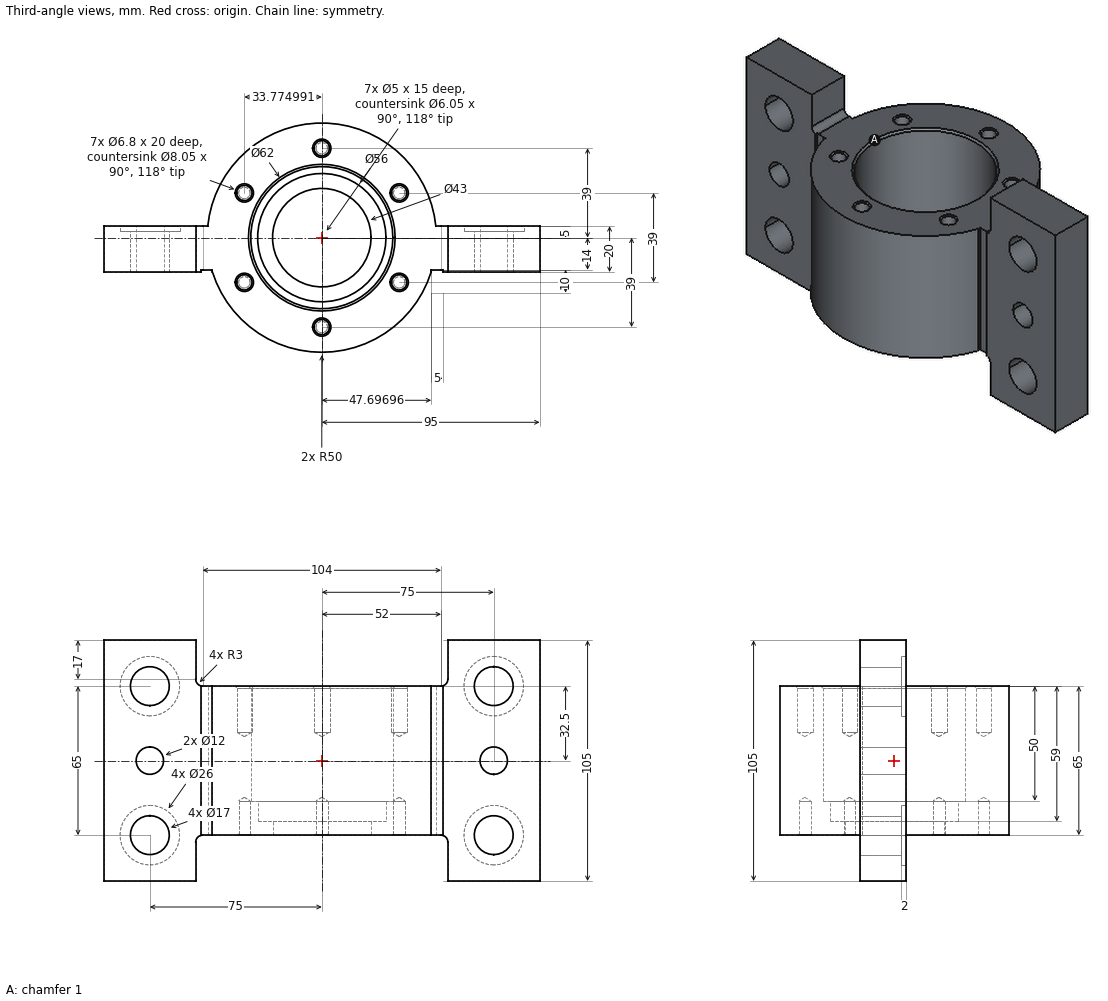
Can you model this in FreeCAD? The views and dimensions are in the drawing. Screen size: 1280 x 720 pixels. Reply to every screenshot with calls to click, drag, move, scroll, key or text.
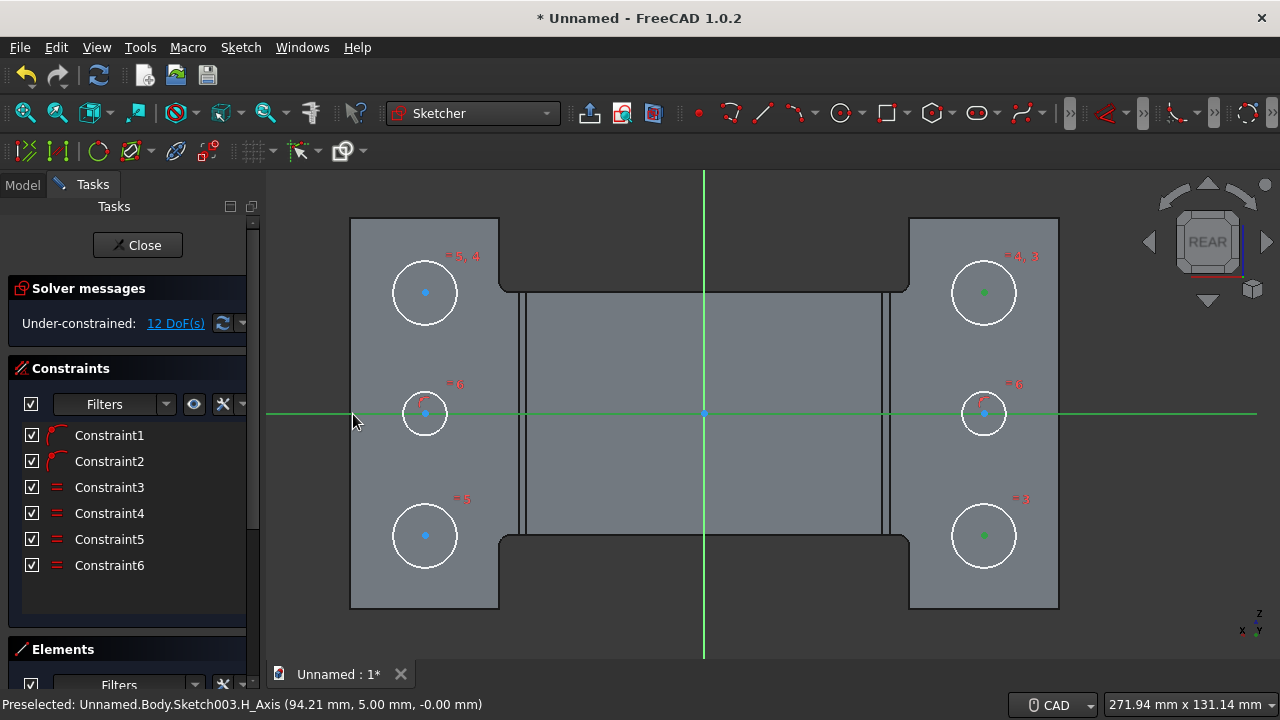
key(s)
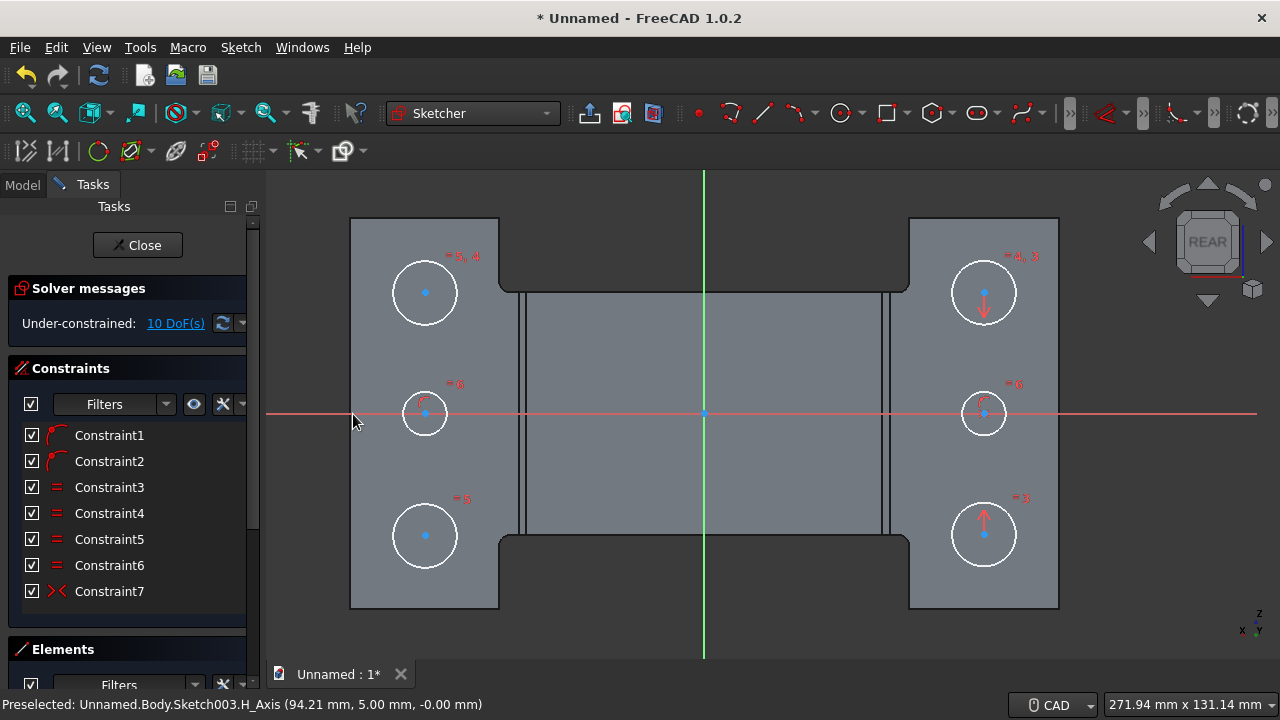
click(984, 293)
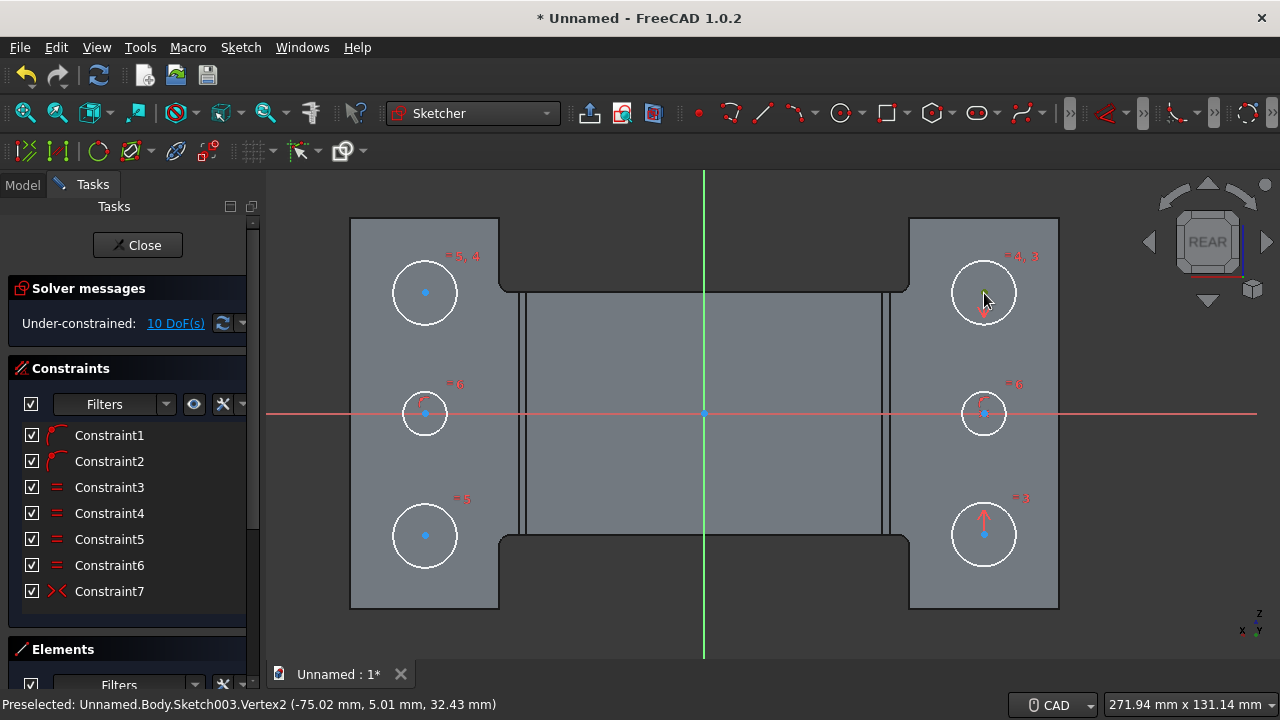
click(425, 293)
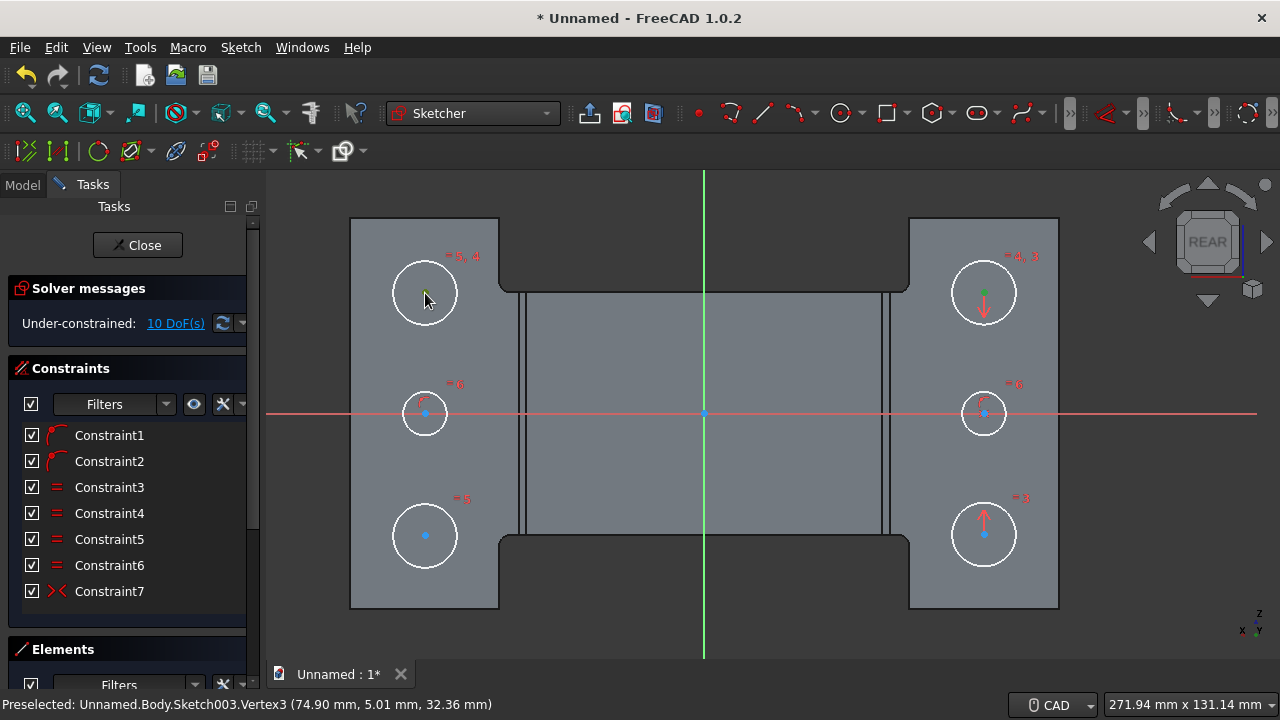
click(704, 600)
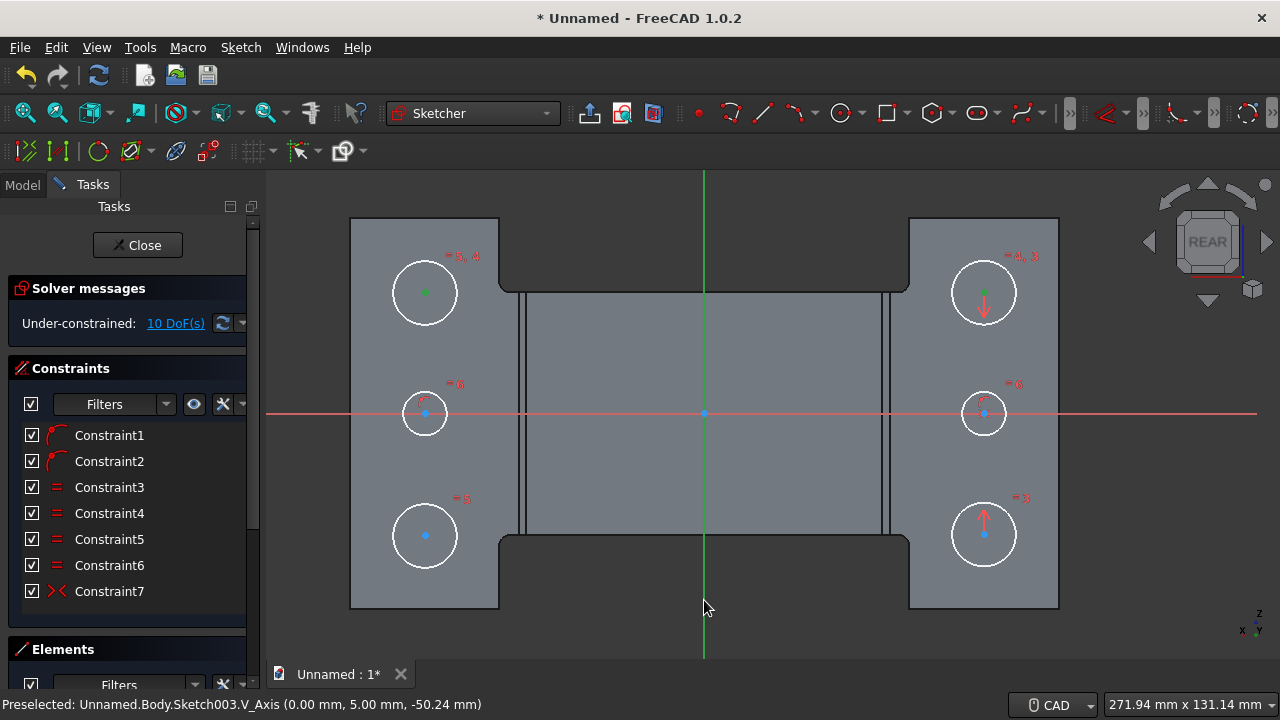
key(s)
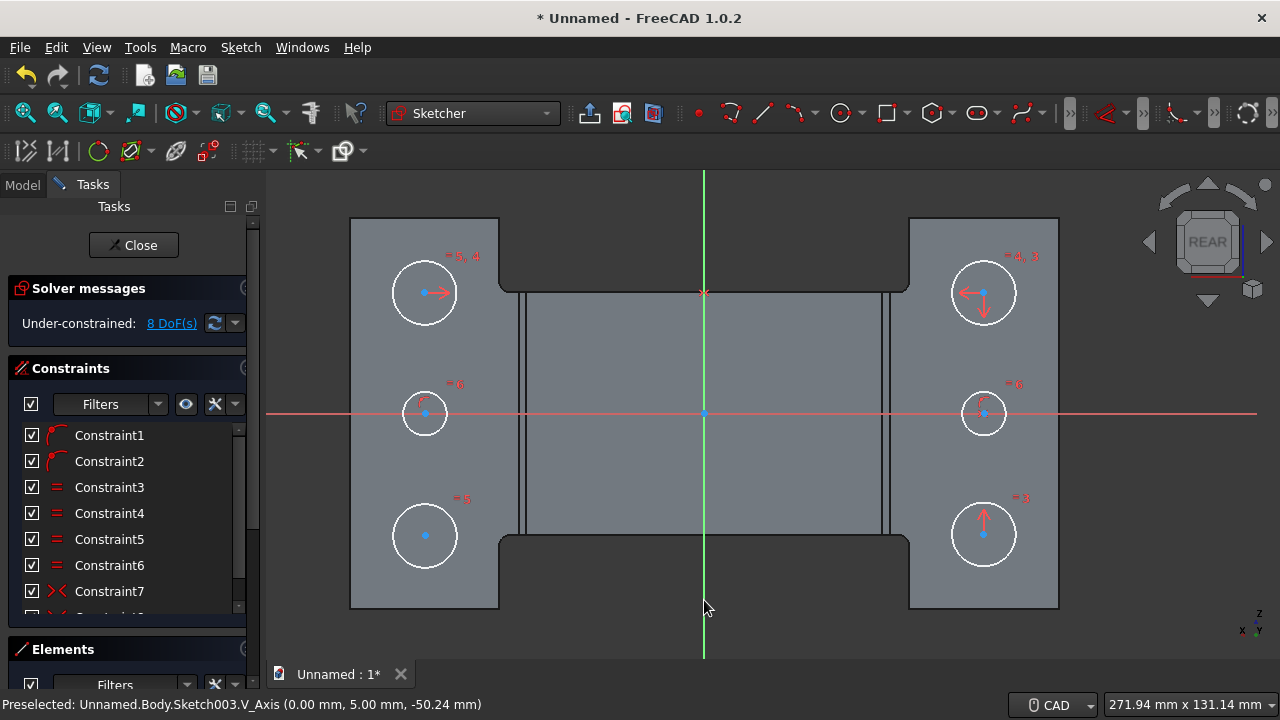
click(984, 534)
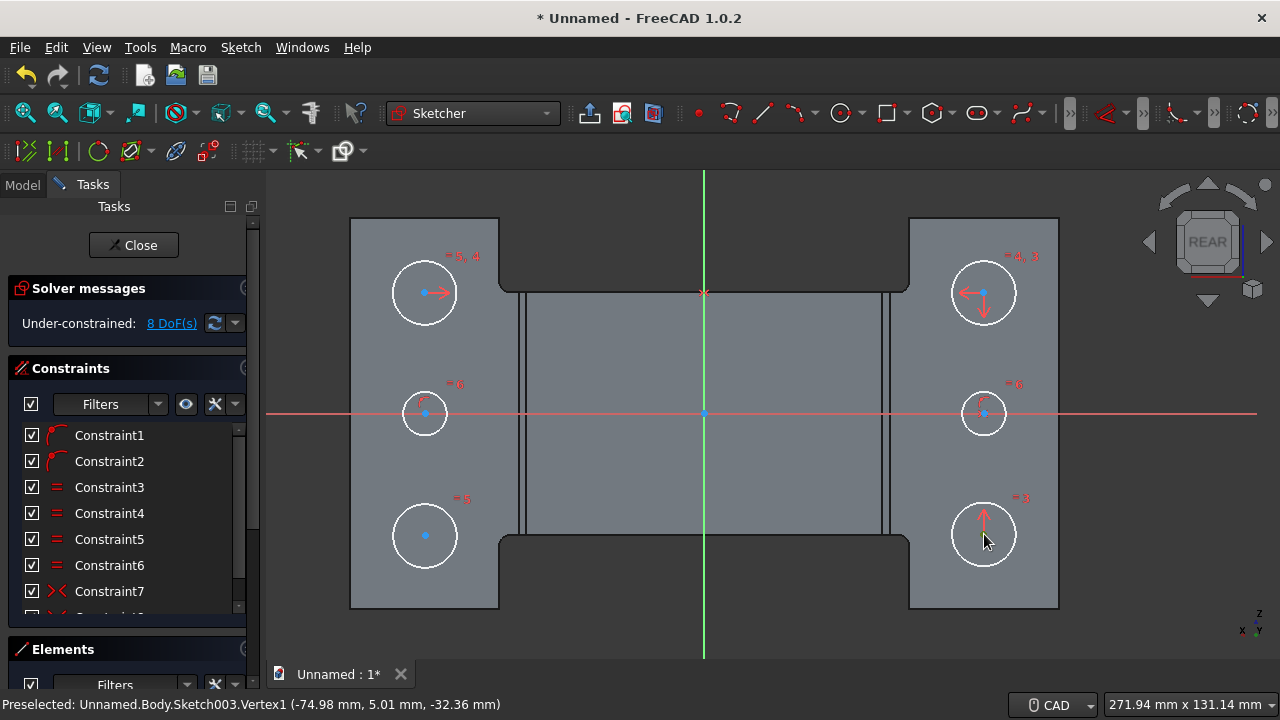
click(425, 536)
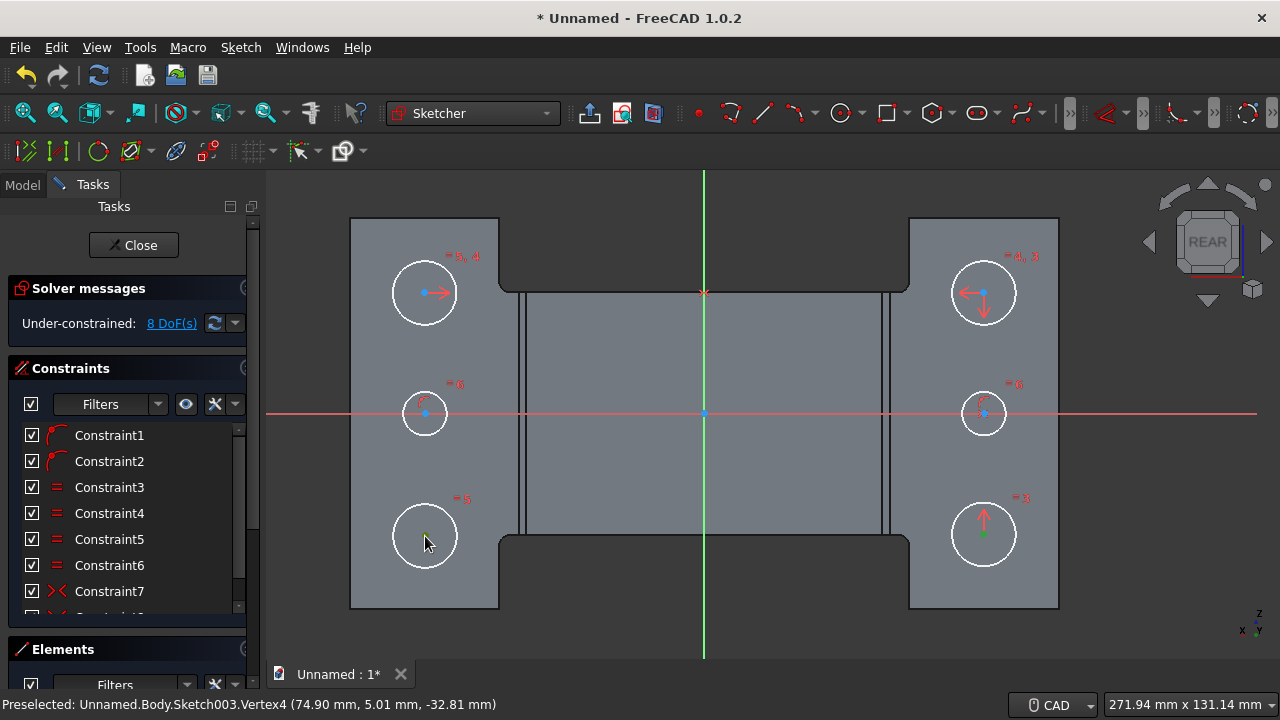
click(704, 600)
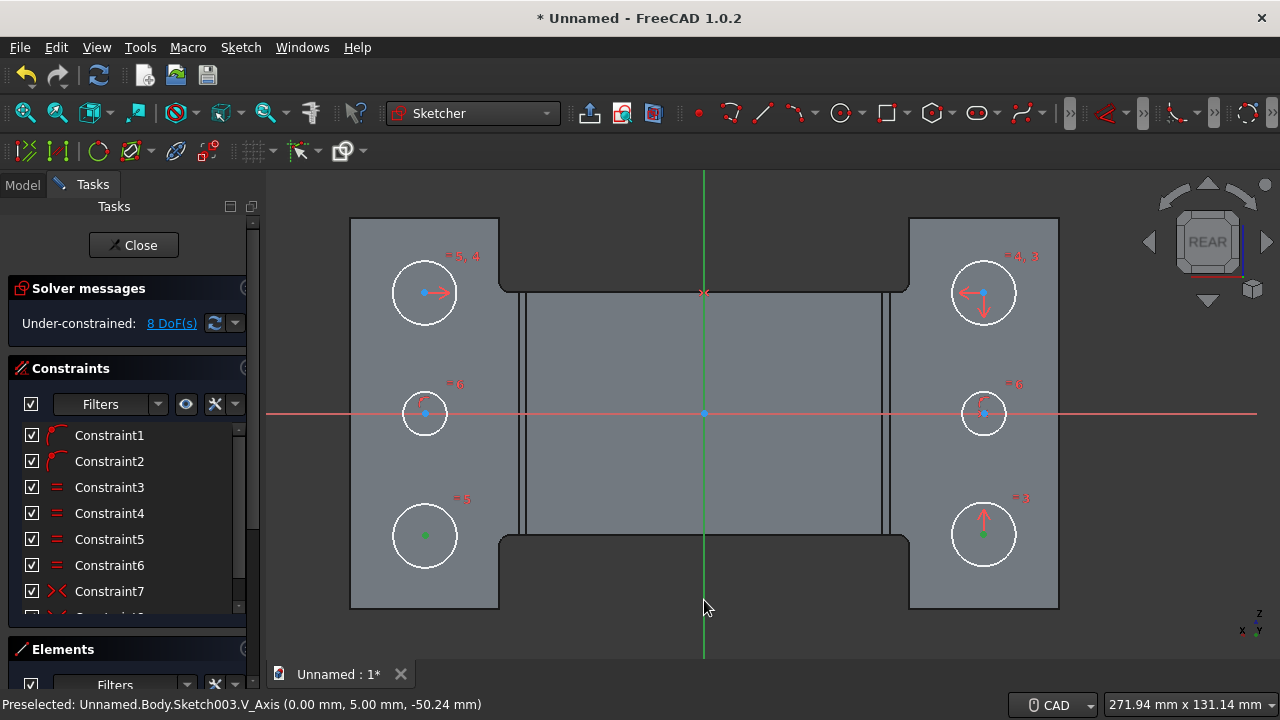
key(s)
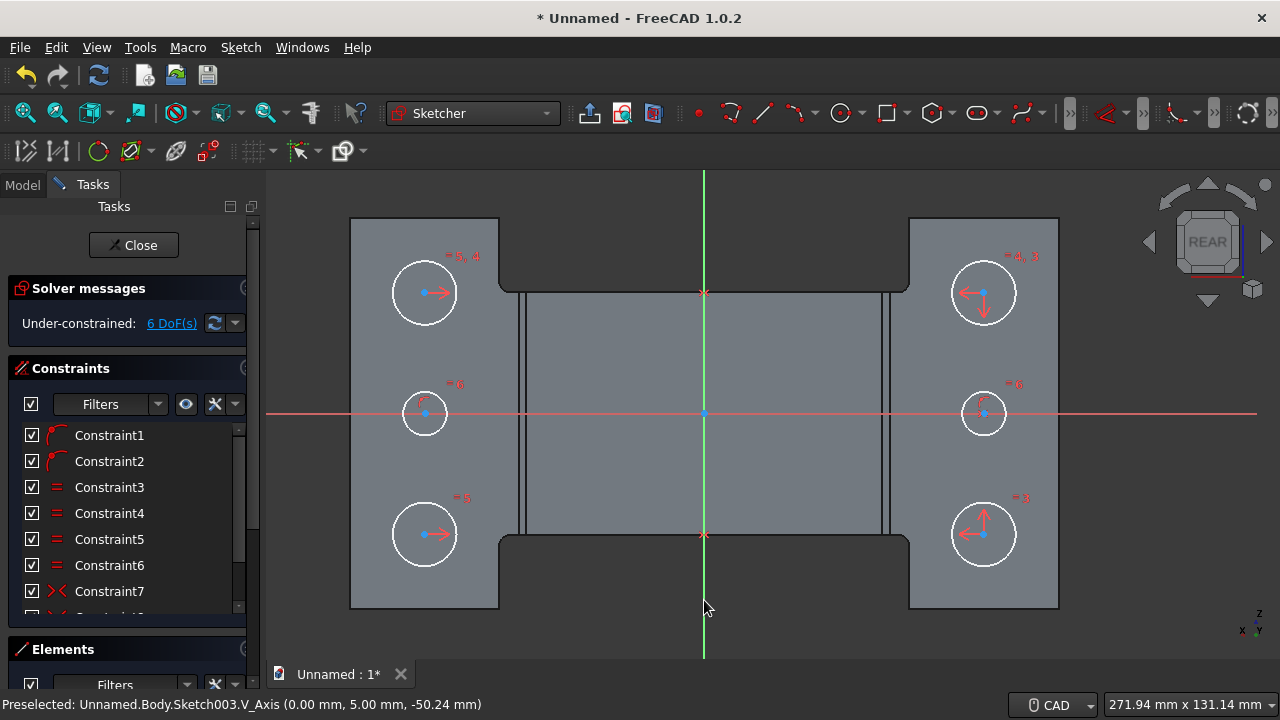
click(1106, 114)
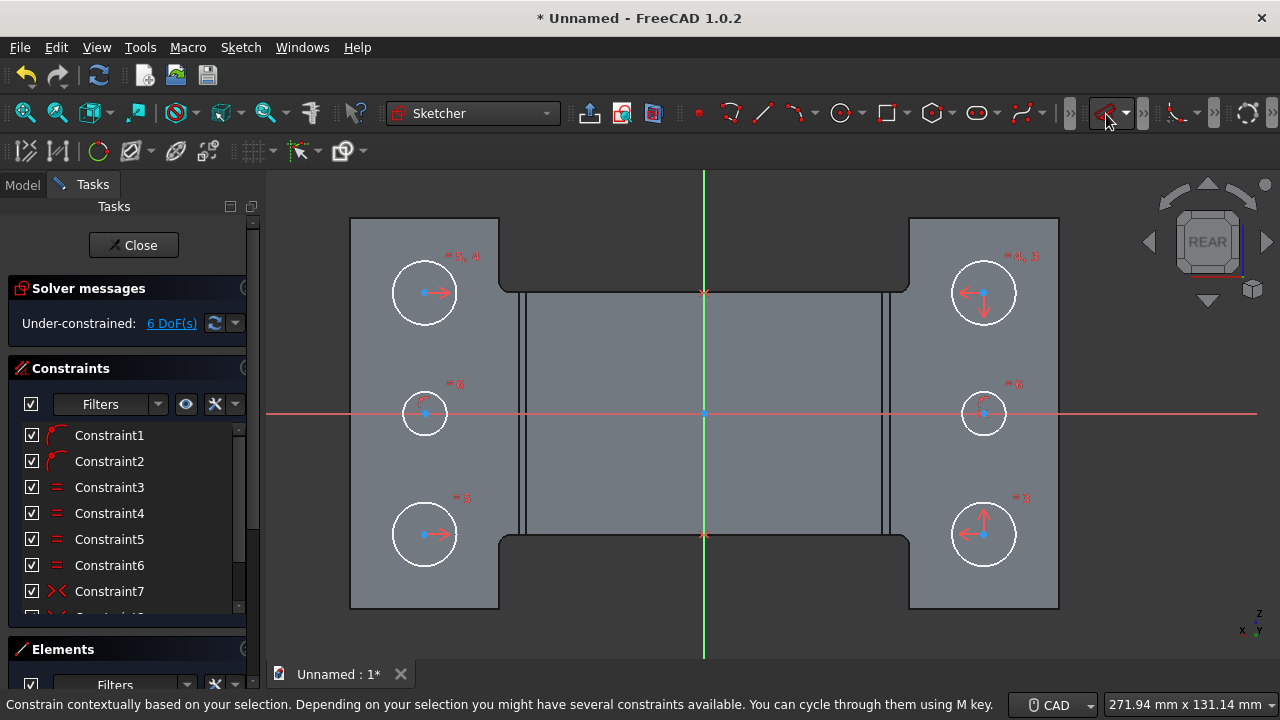
click(1006, 512)
click(1029, 489)